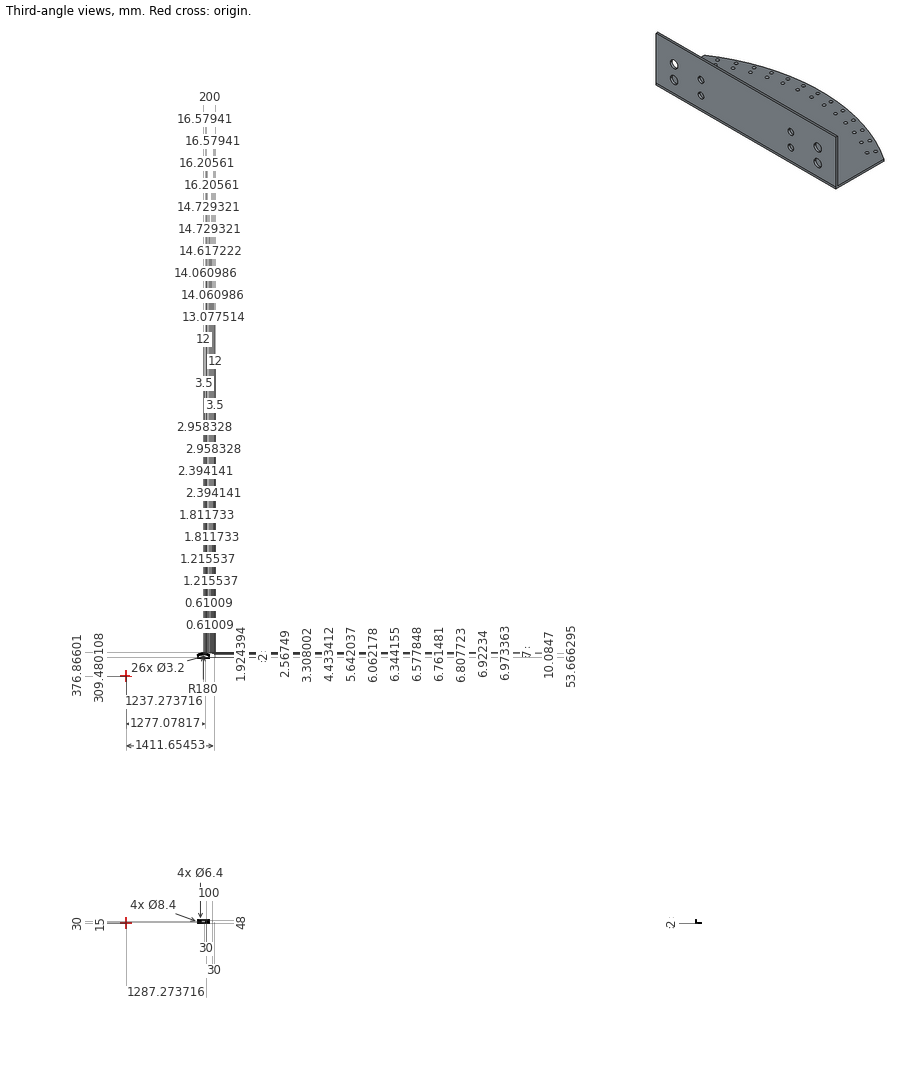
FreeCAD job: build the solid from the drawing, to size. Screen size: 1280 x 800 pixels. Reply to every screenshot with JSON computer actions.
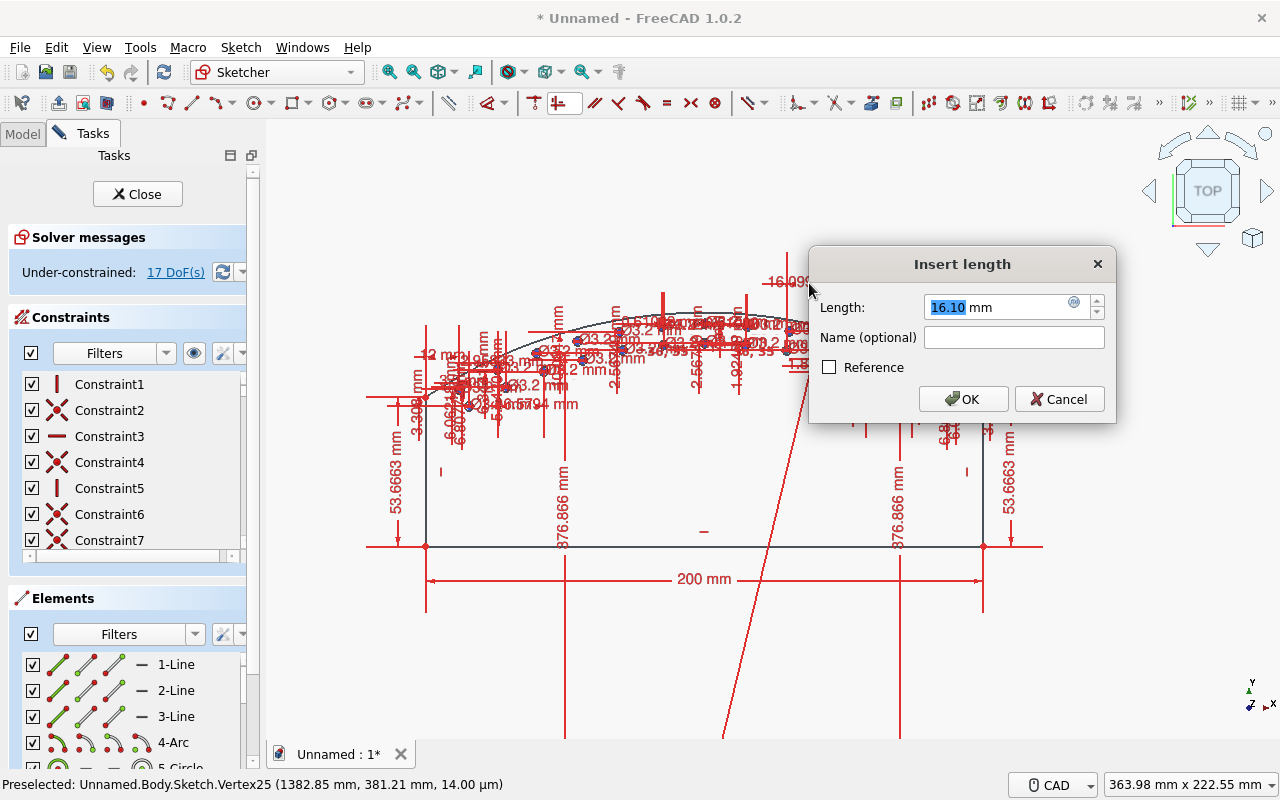
{"action": "type", "text": "16.20561"}
{"action": "key", "text": "Return"}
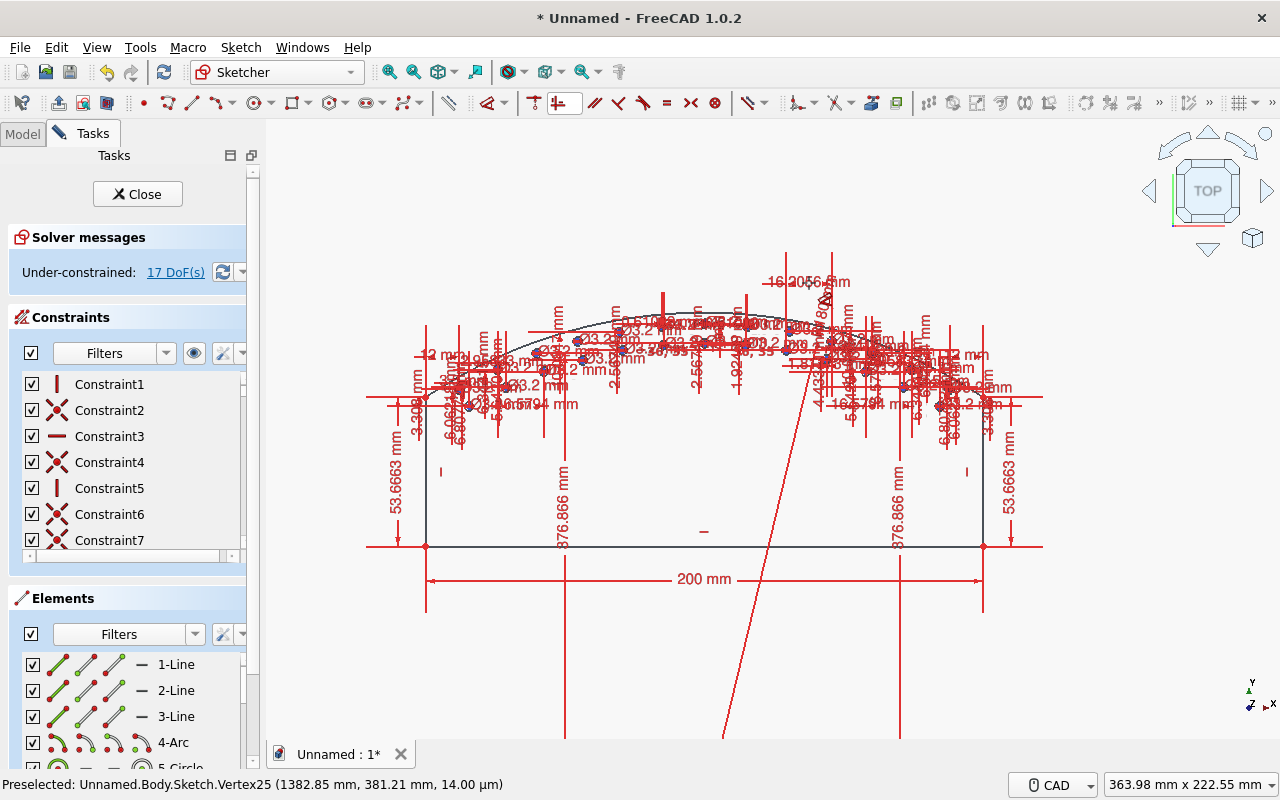
{"action": "scroll", "coordinate": [827, 359], "scroll_direction": "up", "scroll_amount": 4}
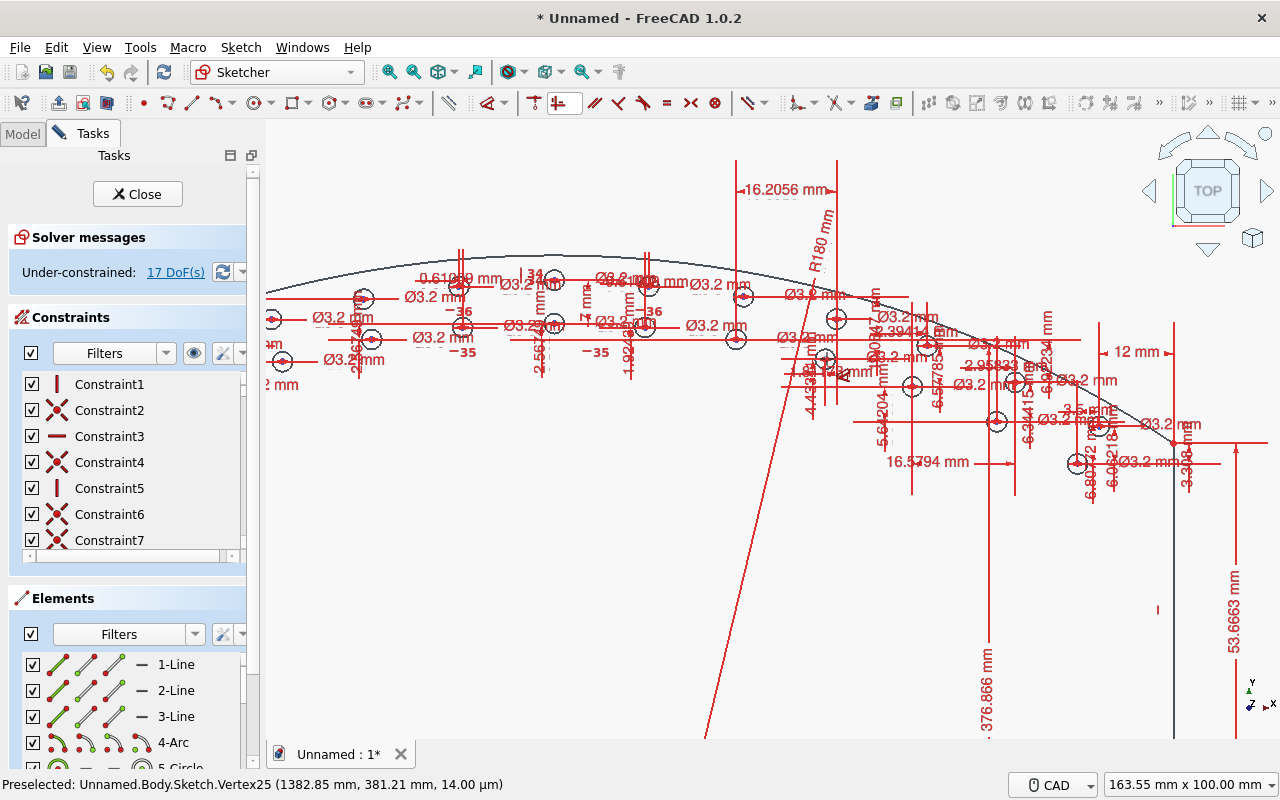
{"action": "left_click", "coordinate": [825, 359]}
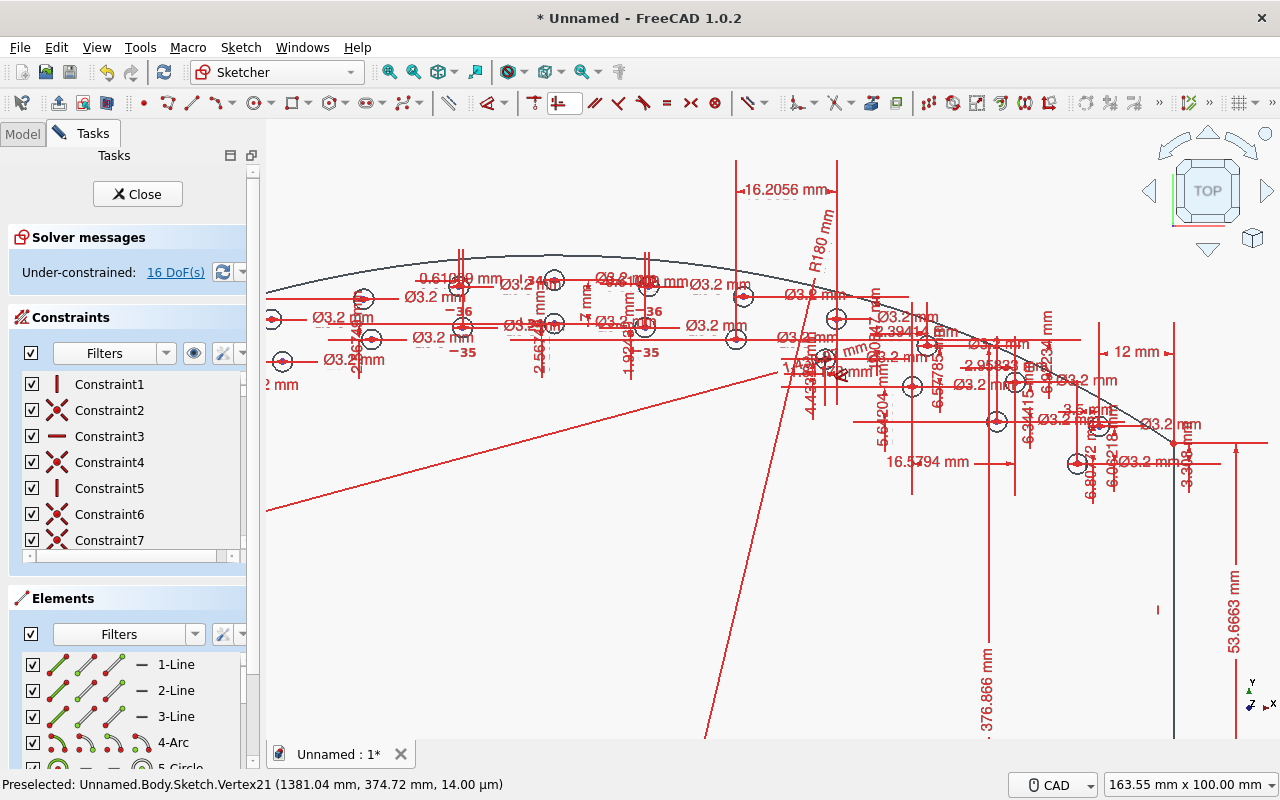
{"action": "left_click", "coordinate": [837, 319]}
{"action": "left_click", "coordinate": [791, 339]}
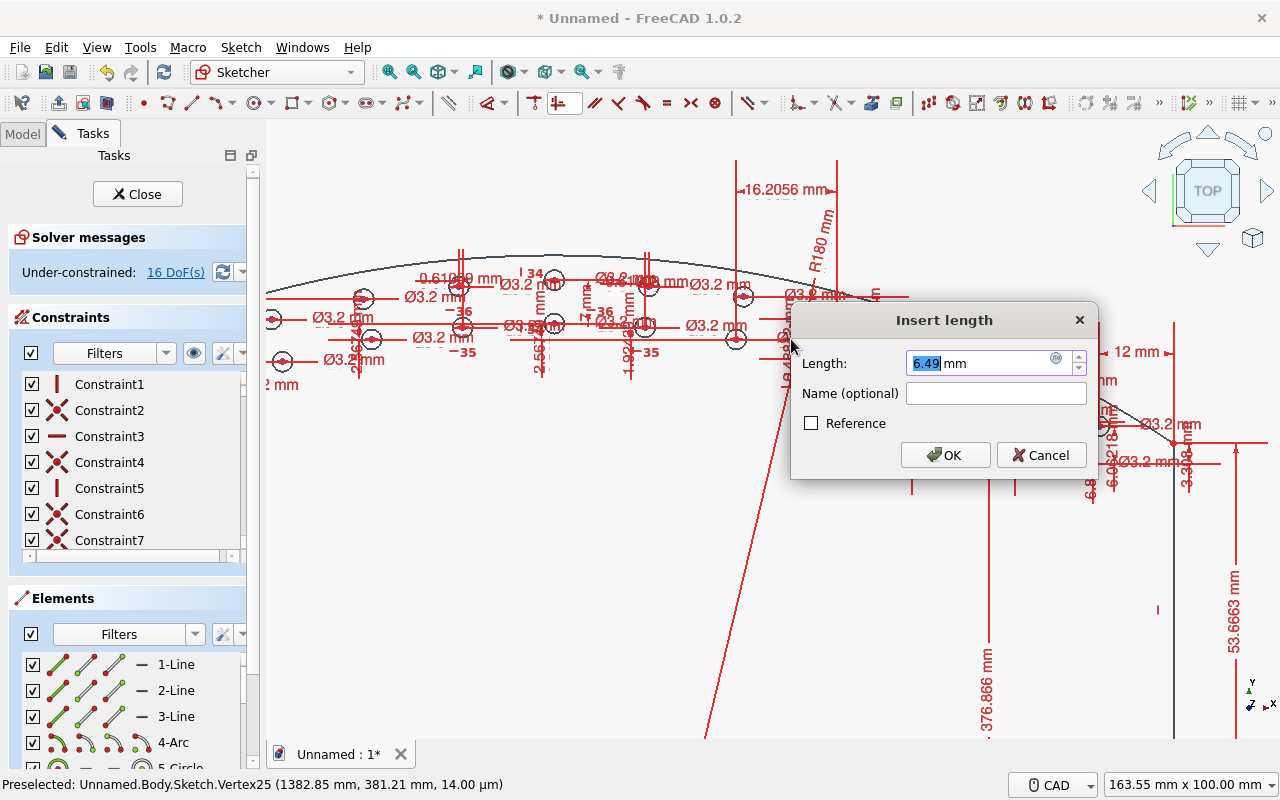
{"action": "type", "text": "6.761481"}
{"action": "key", "text": "Return"}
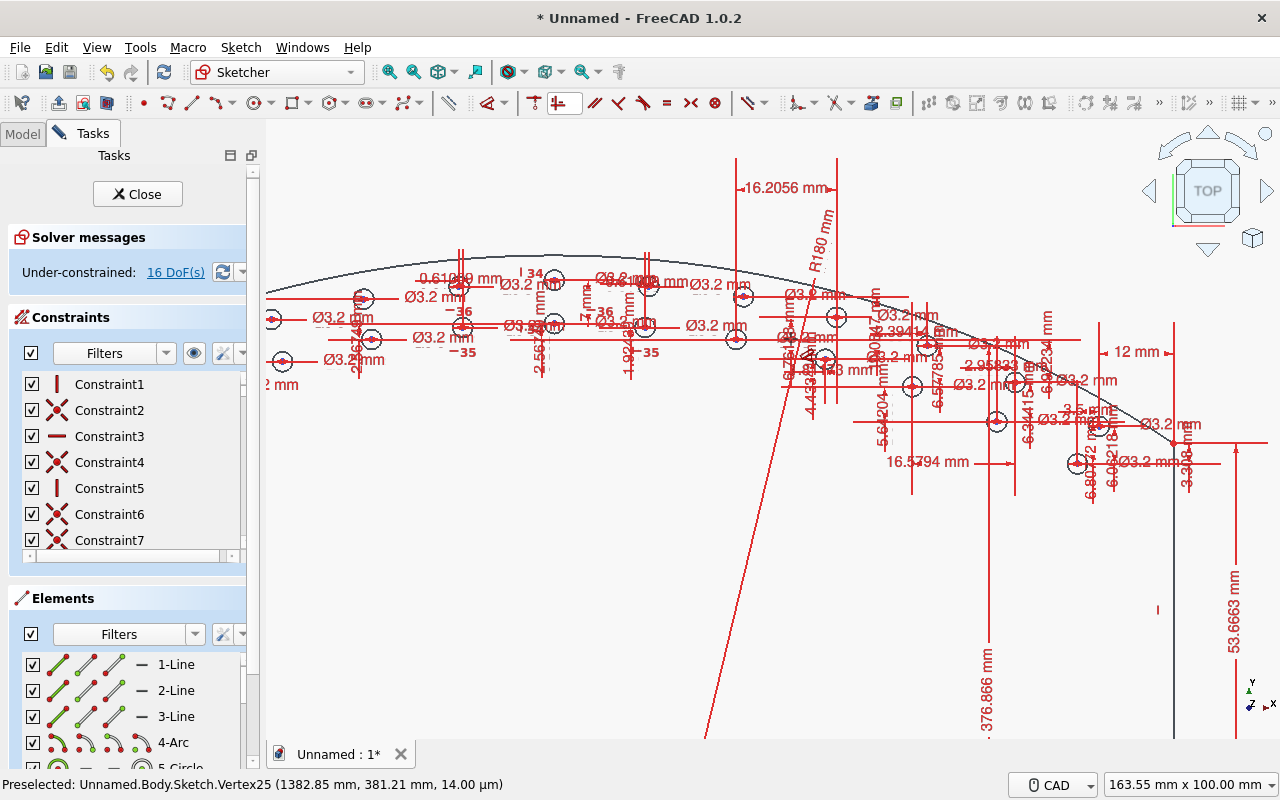
{"action": "scroll", "coordinate": [736, 340], "scroll_direction": "up", "scroll_amount": 9}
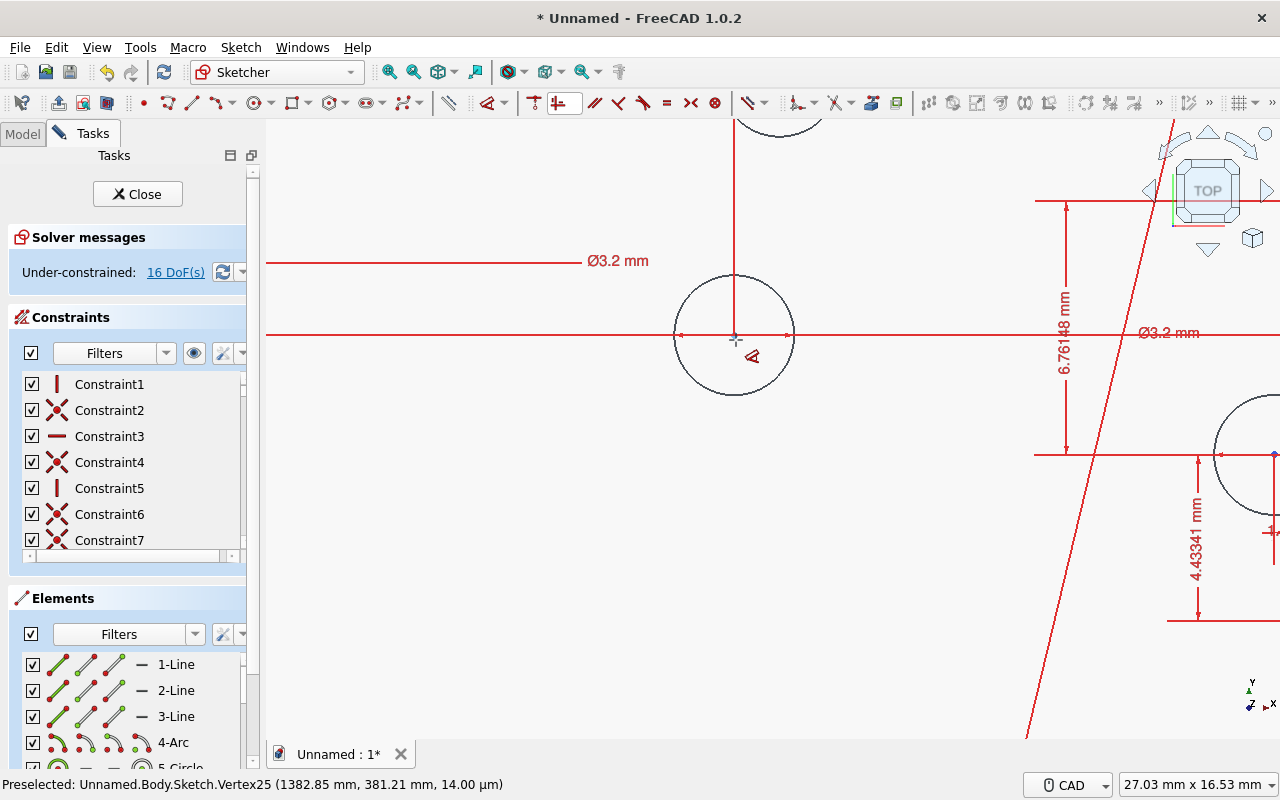
{"action": "left_click", "coordinate": [734, 335]}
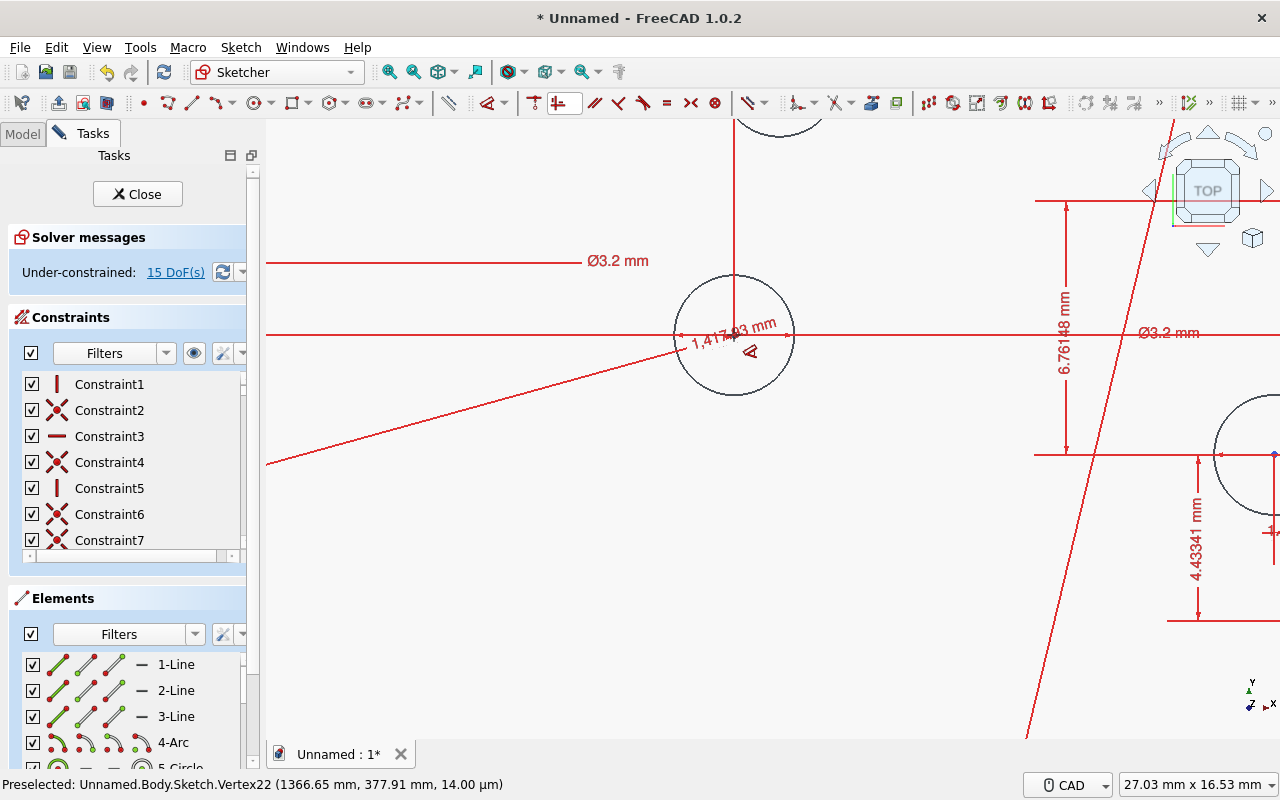
{"action": "scroll", "coordinate": [791, 351], "scroll_direction": "down", "scroll_amount": 13}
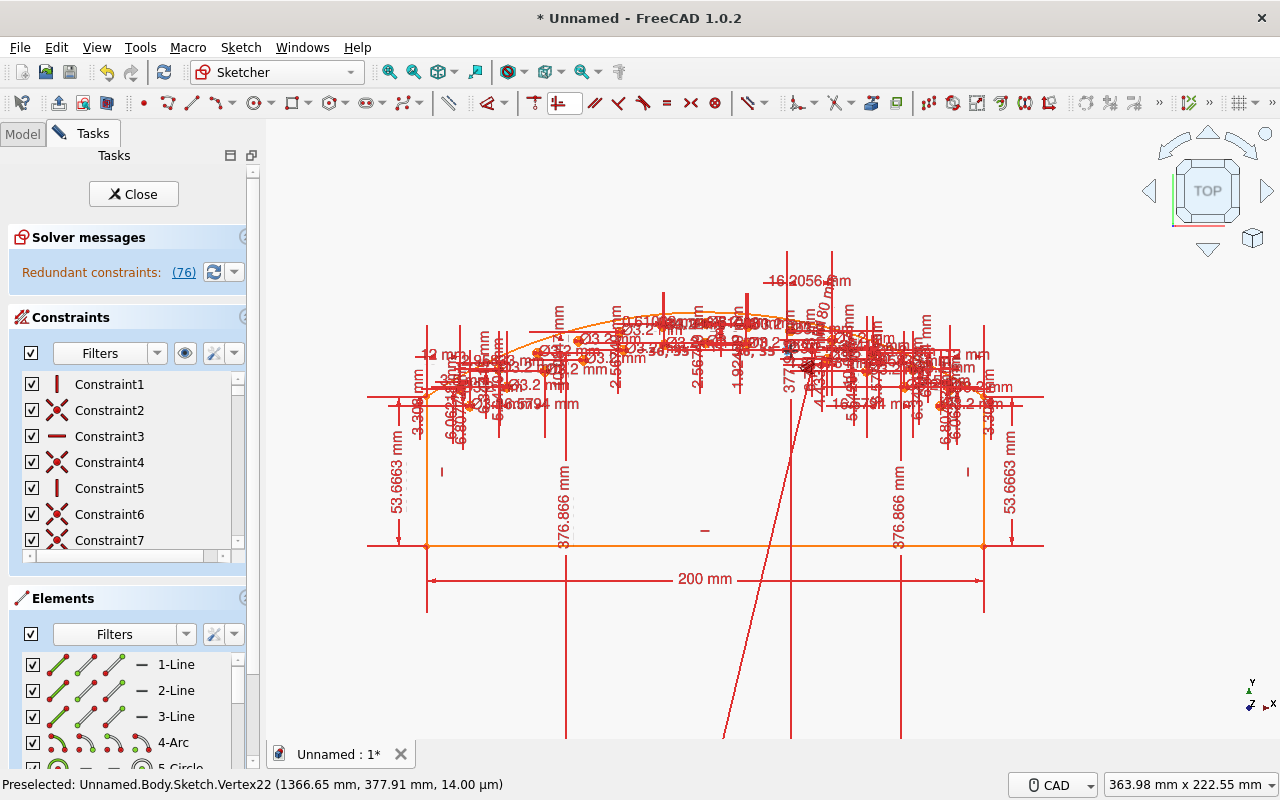
{"action": "scroll", "coordinate": [791, 331], "scroll_direction": "up", "scroll_amount": 13}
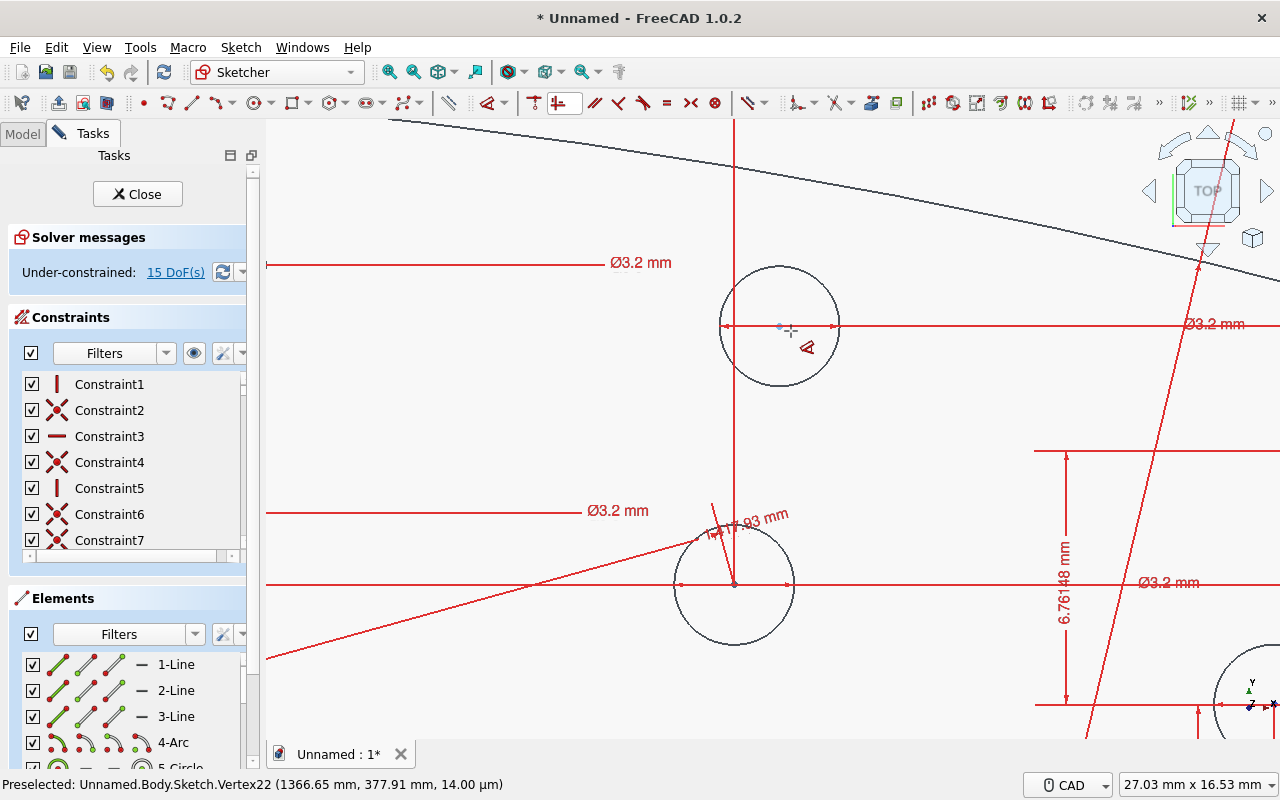
{"action": "left_click", "coordinate": [780, 326]}
{"action": "left_click", "coordinate": [757, 292]}